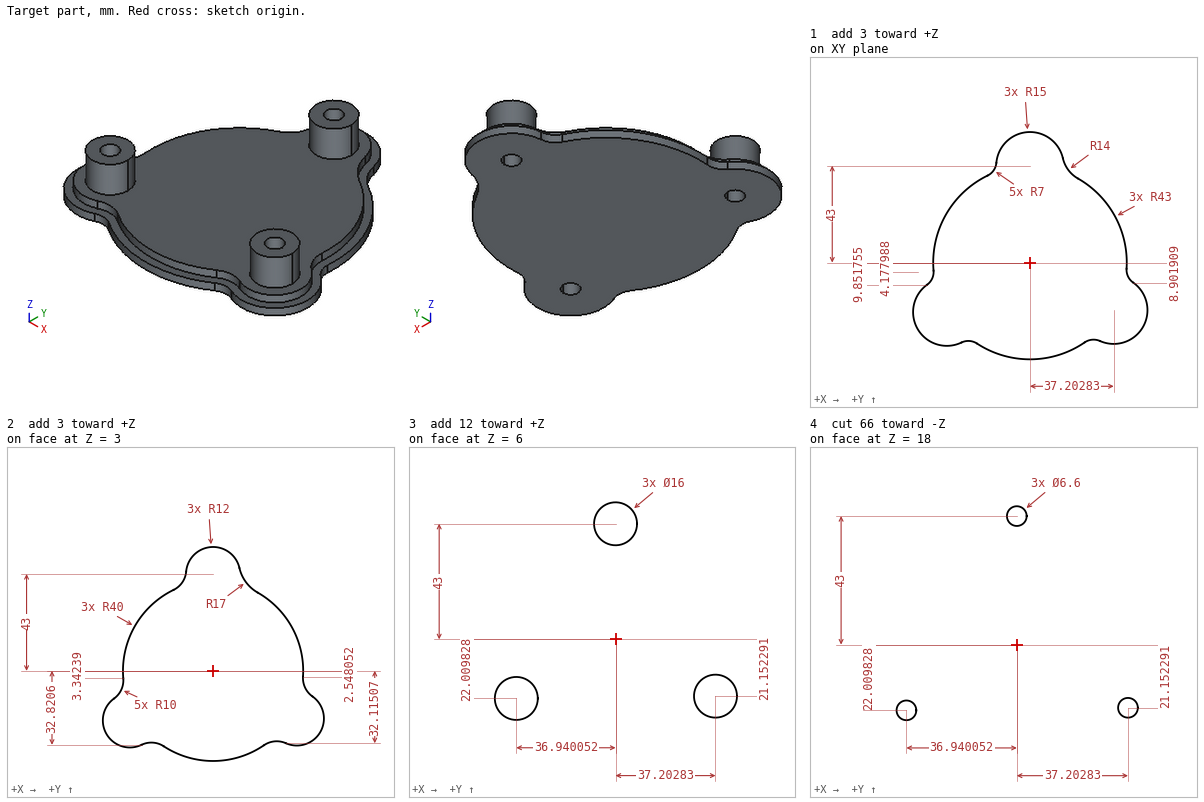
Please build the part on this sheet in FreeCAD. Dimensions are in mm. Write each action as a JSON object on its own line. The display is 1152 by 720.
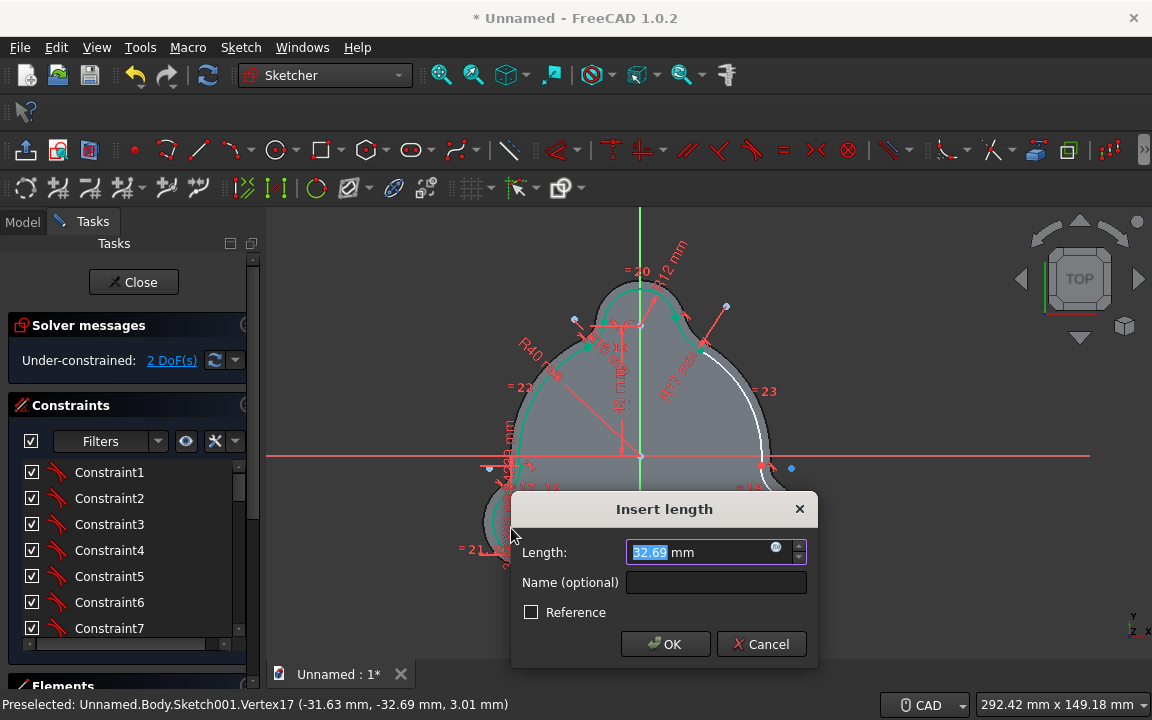
{"action": "type", "text": "32.8206"}
{"action": "key", "text": "Return"}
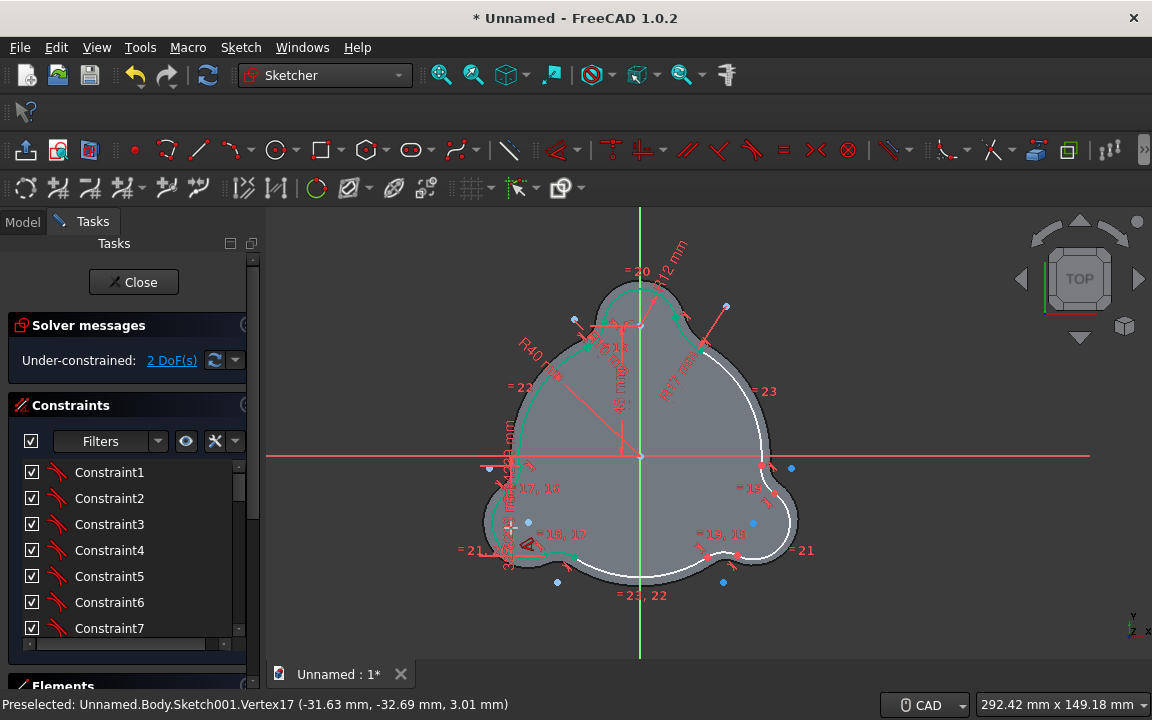
{"action": "left_click", "coordinate": [737, 556]}
{"action": "left_click", "coordinate": [771, 529]}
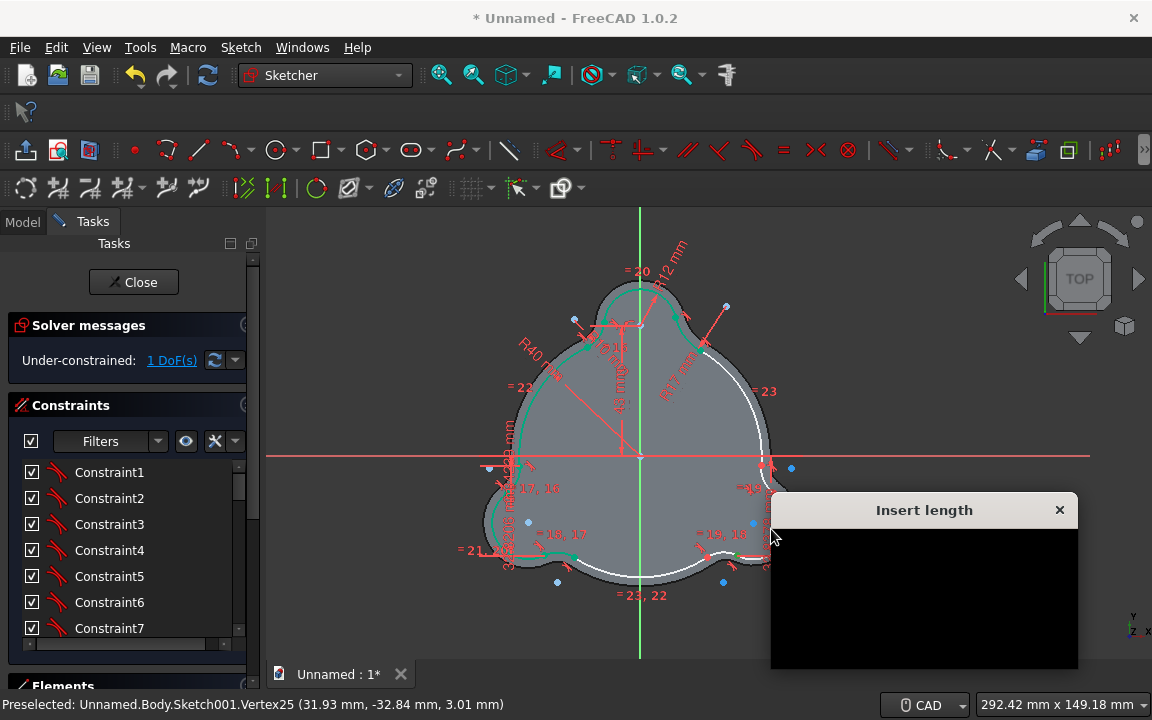
{"action": "type", "text": "32.11507"}
{"action": "key", "text": "Return"}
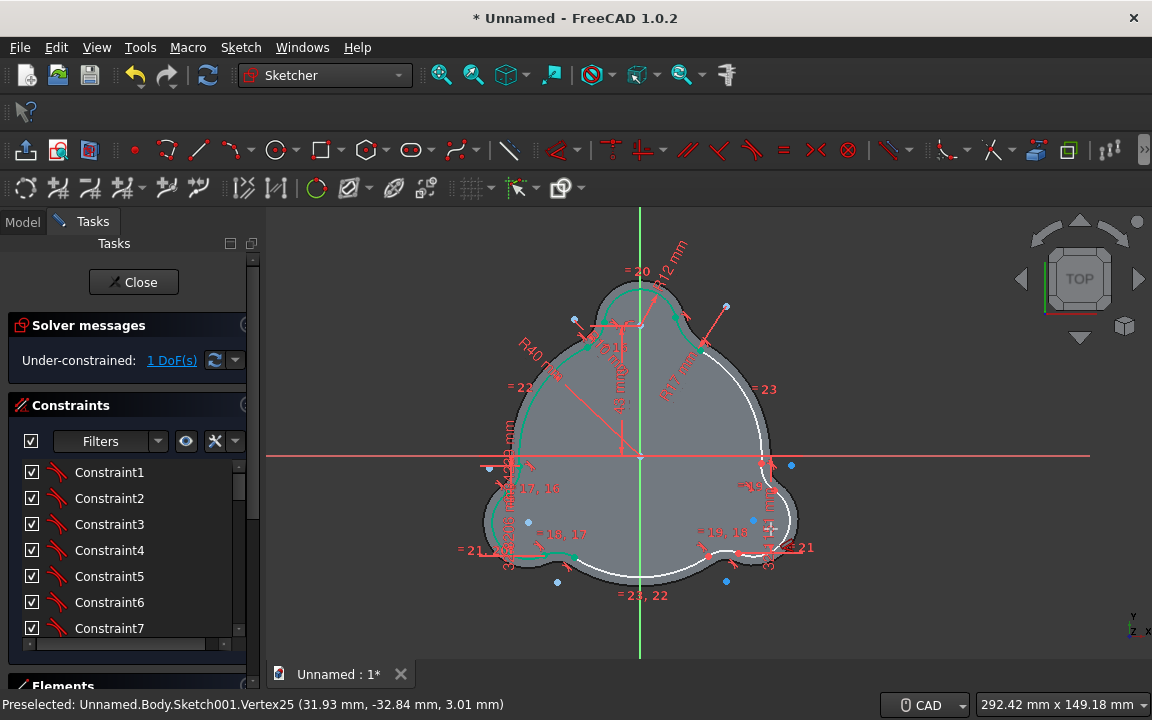
{"action": "scroll", "coordinate": [761, 464], "scroll_direction": "up", "scroll_amount": 9}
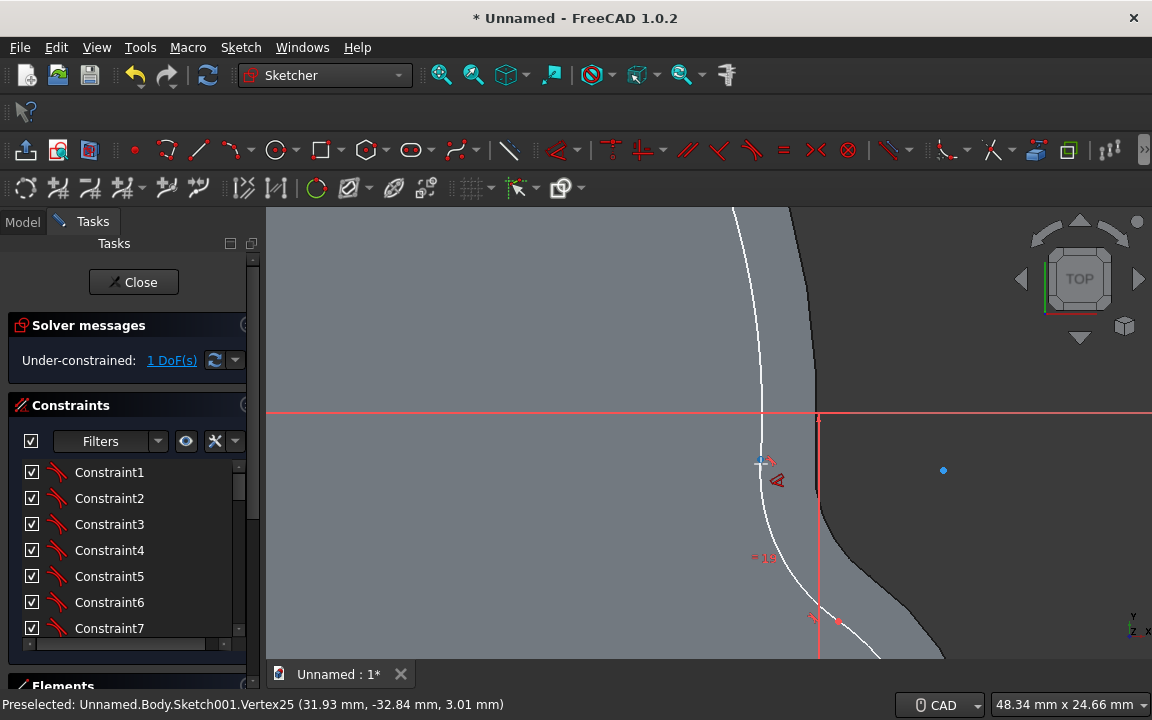
{"action": "left_click", "coordinate": [761, 459]}
{"action": "left_click", "coordinate": [795, 436]}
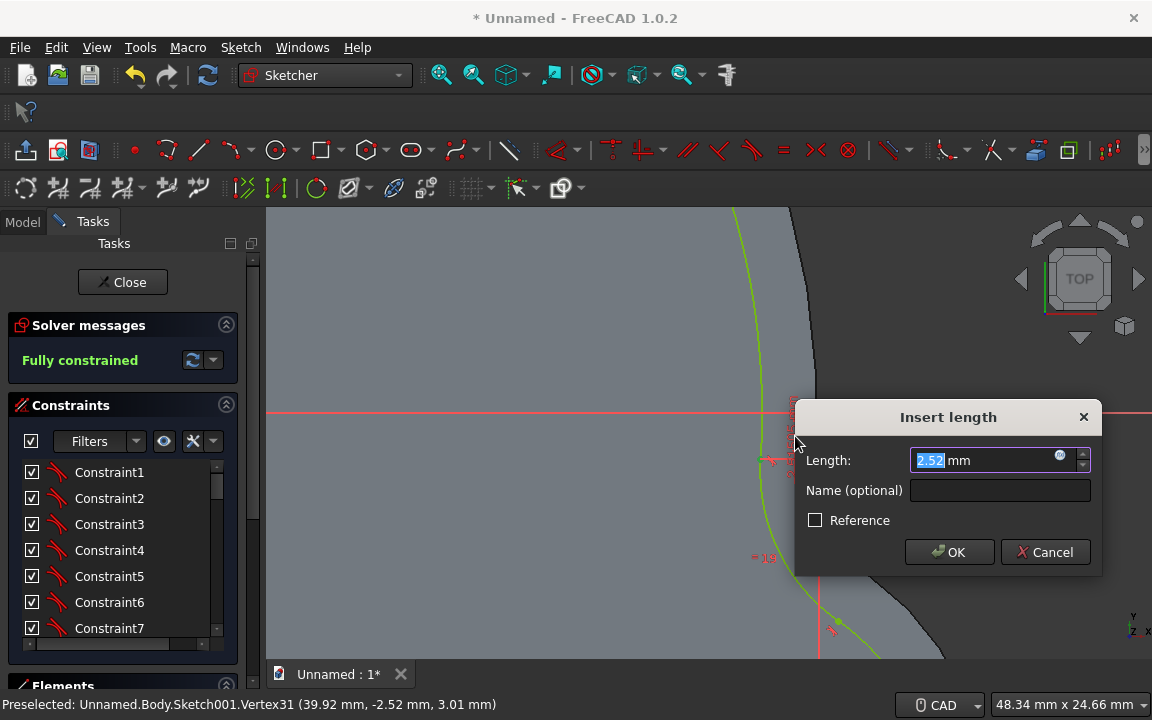
{"action": "type", "text": "2.548052"}
{"action": "key", "text": "Return"}
{"action": "key", "text": "Escape"}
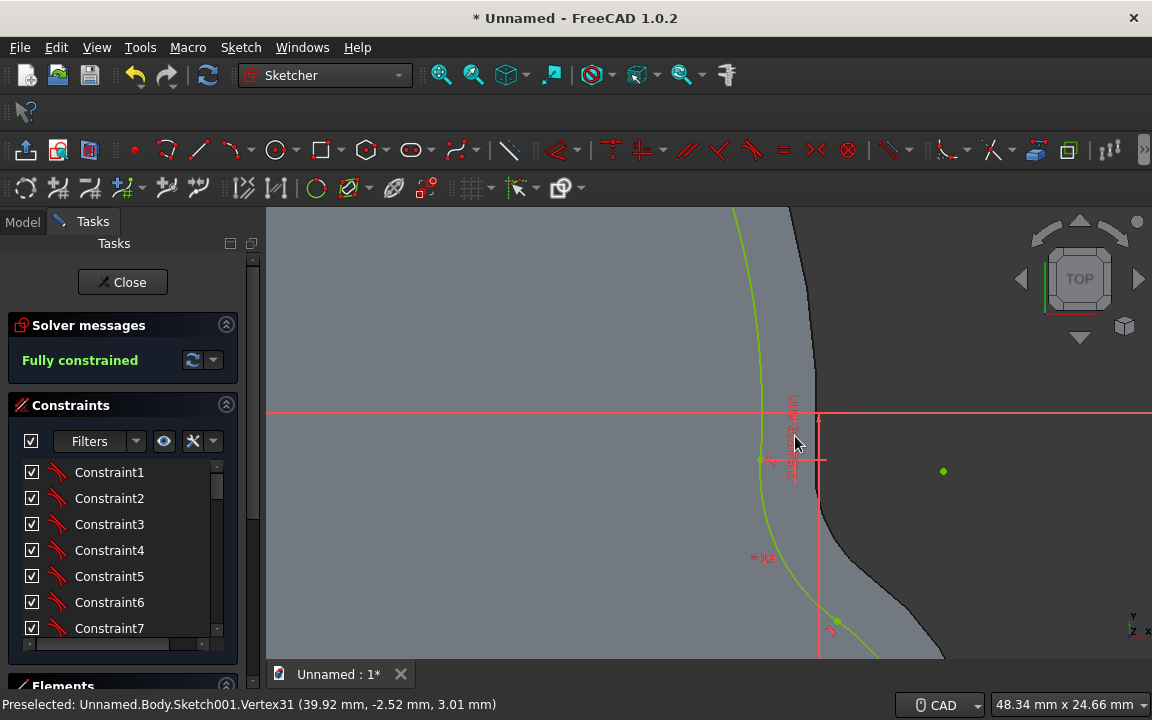
{"action": "left_click", "coordinate": [123, 282]}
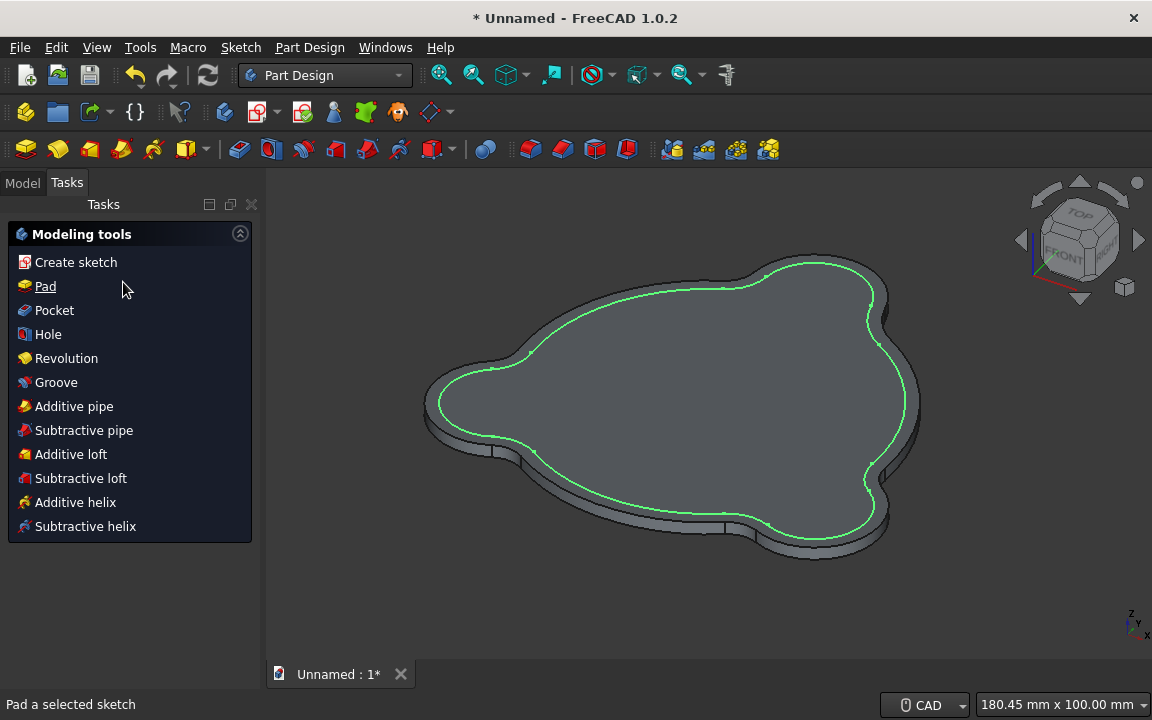
{"action": "left_click", "coordinate": [26, 150]}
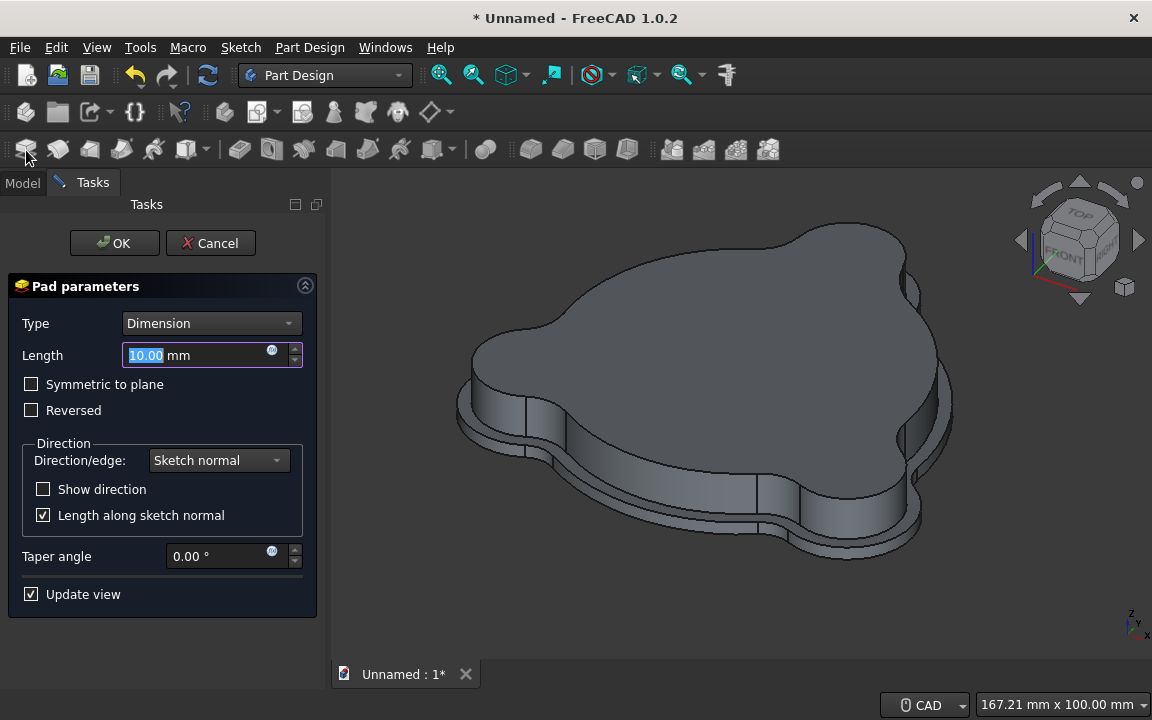
{"action": "type", "text": "3"}
{"action": "key", "text": "Tab"}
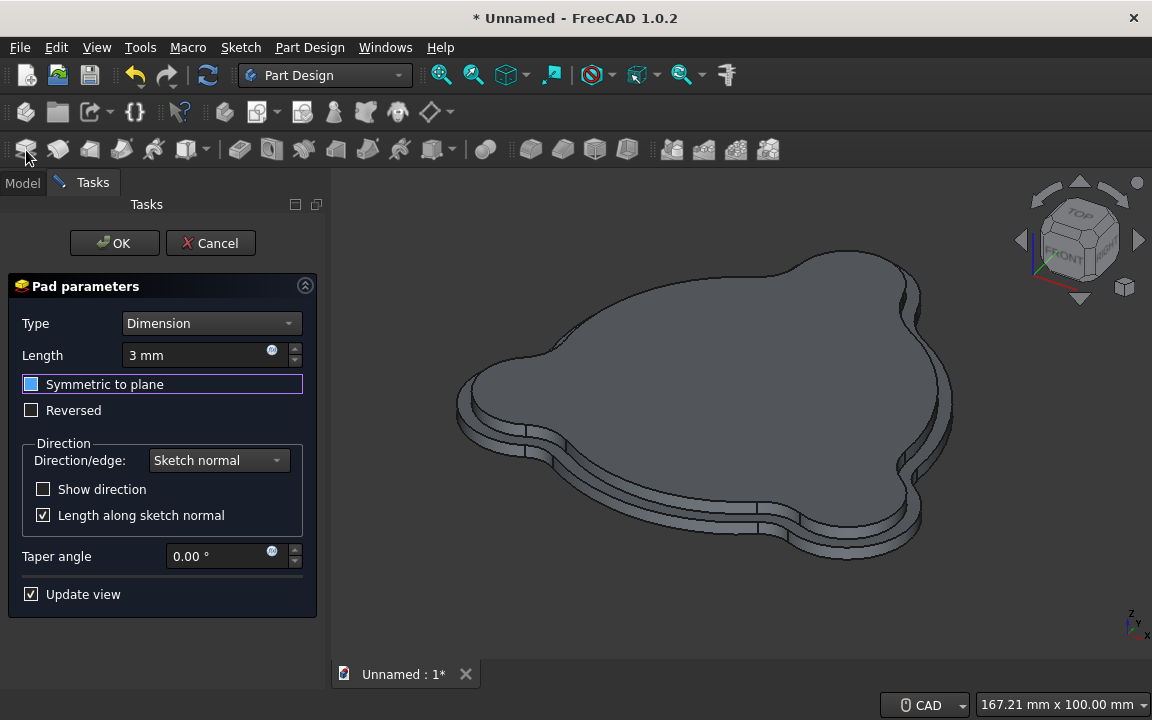
{"action": "left_click", "coordinate": [115, 243]}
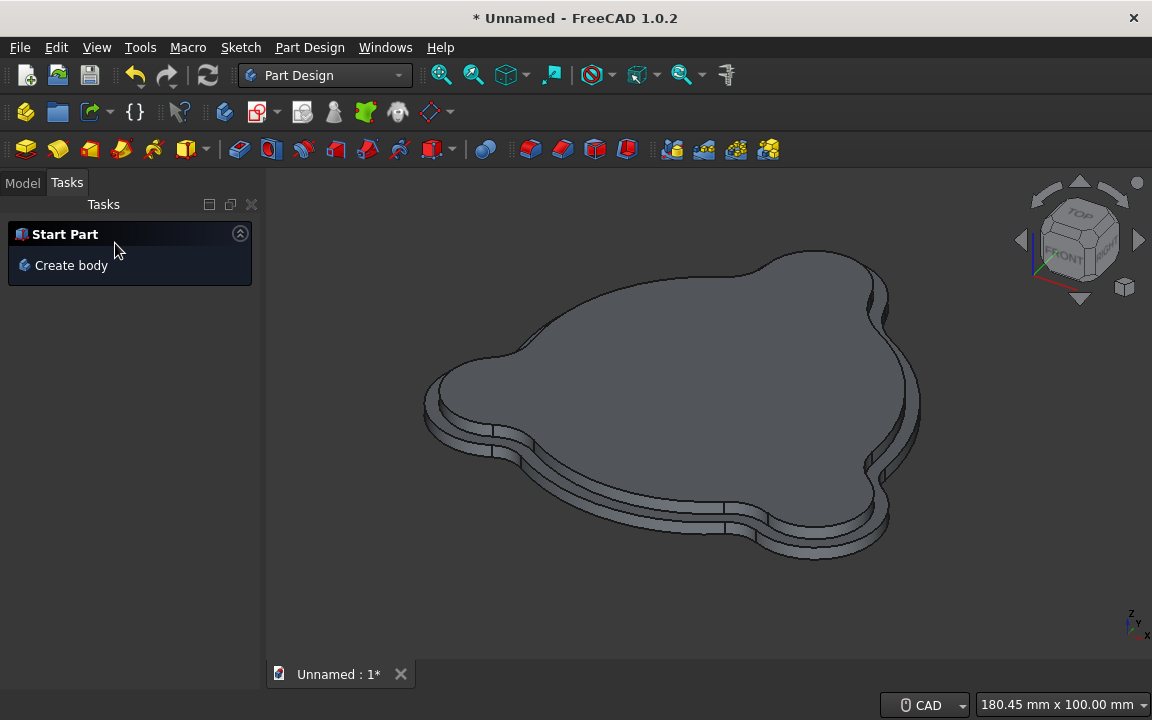
{"action": "left_click", "coordinate": [695, 403]}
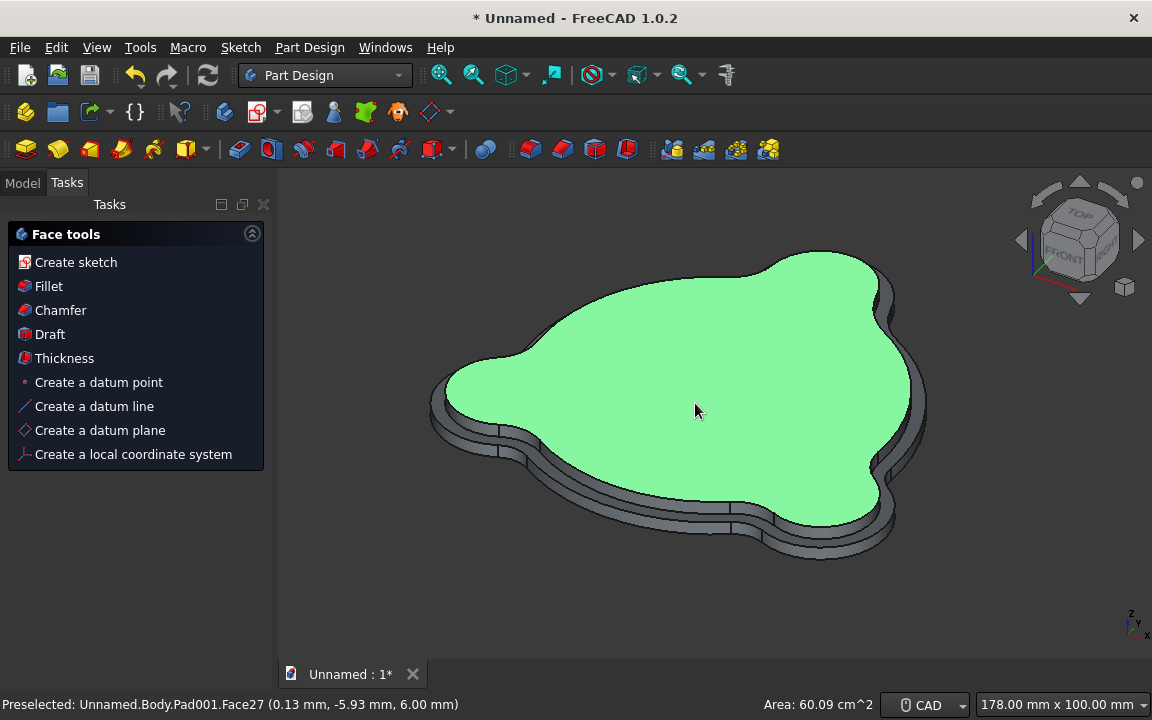
{"action": "left_click", "coordinate": [258, 112]}